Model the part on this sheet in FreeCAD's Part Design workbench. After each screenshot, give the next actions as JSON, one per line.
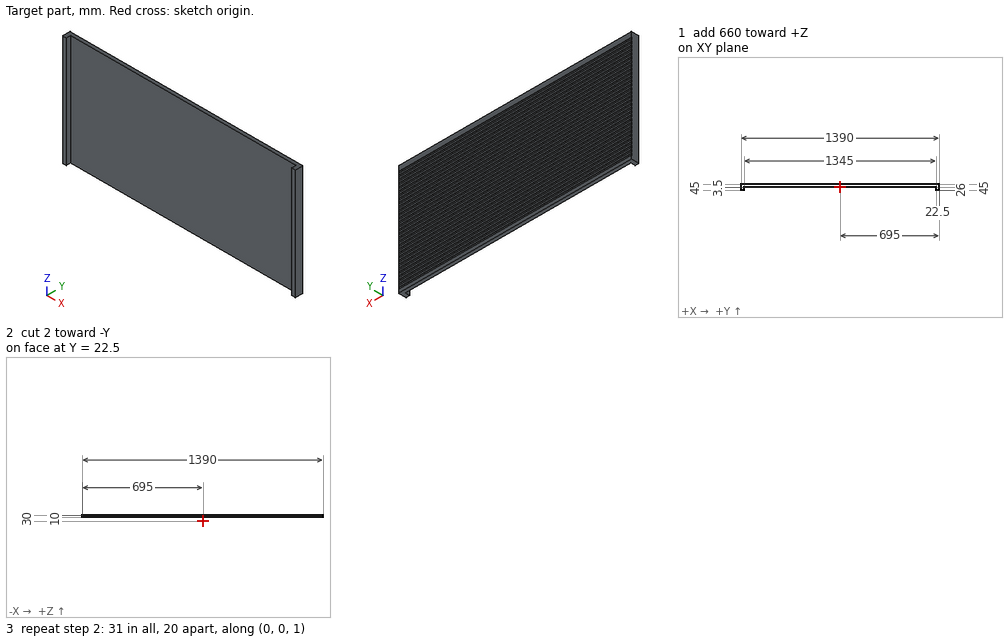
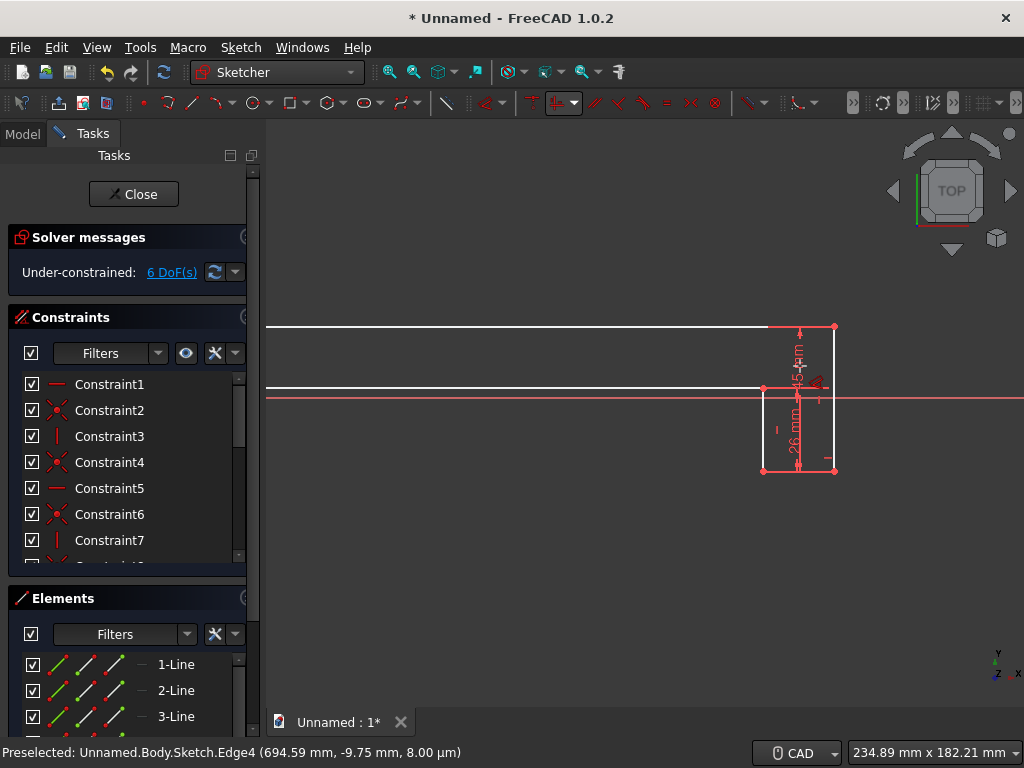
{"action": "scroll", "coordinate": [774, 415], "scroll_direction": "down", "scroll_amount": 12}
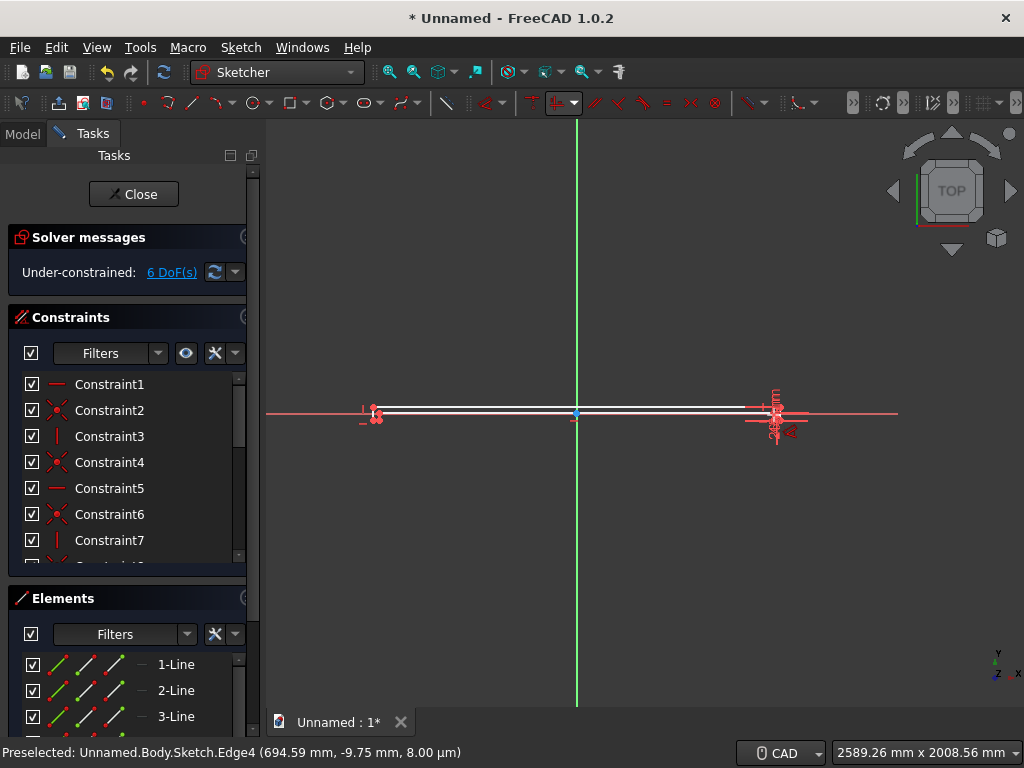
{"action": "scroll", "coordinate": [373, 411], "scroll_direction": "up", "scroll_amount": 9}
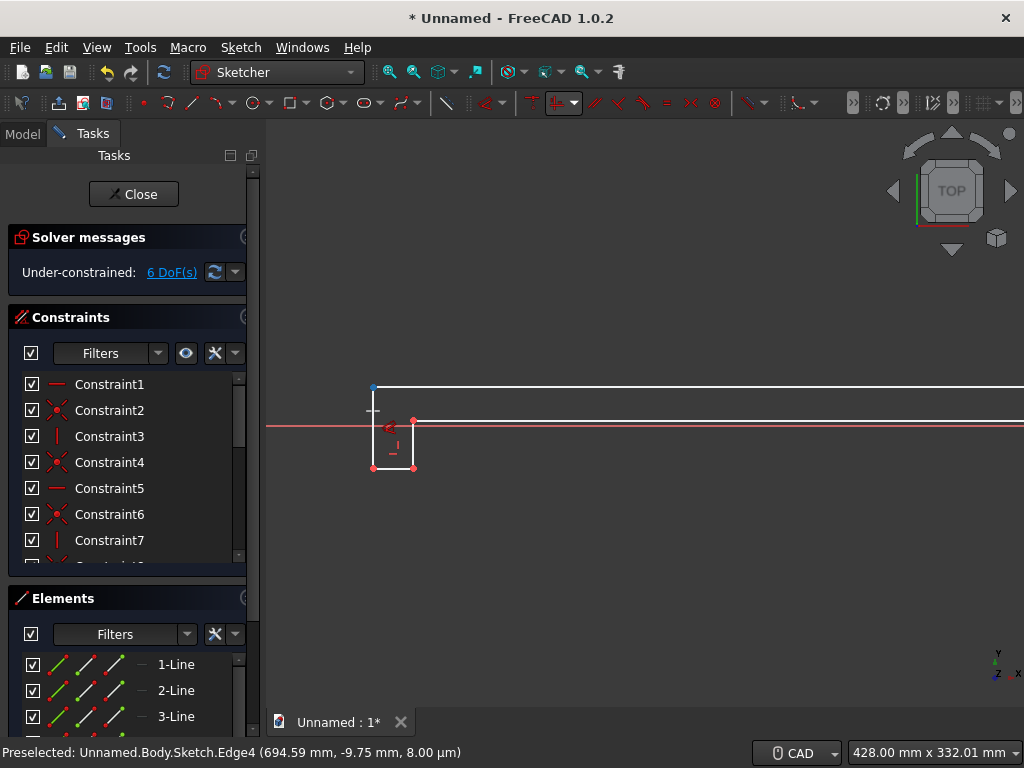
{"action": "left_click", "coordinate": [373, 412]}
{"action": "left_click", "coordinate": [339, 409]}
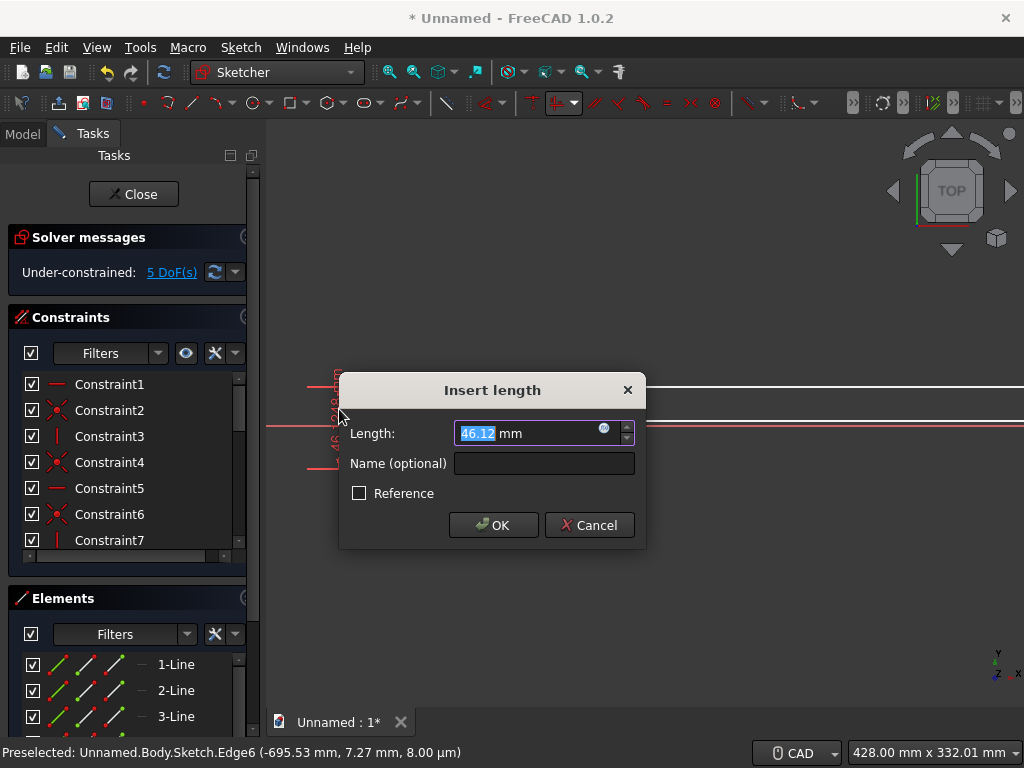
{"action": "type", "text": "45"}
{"action": "key", "text": "Return"}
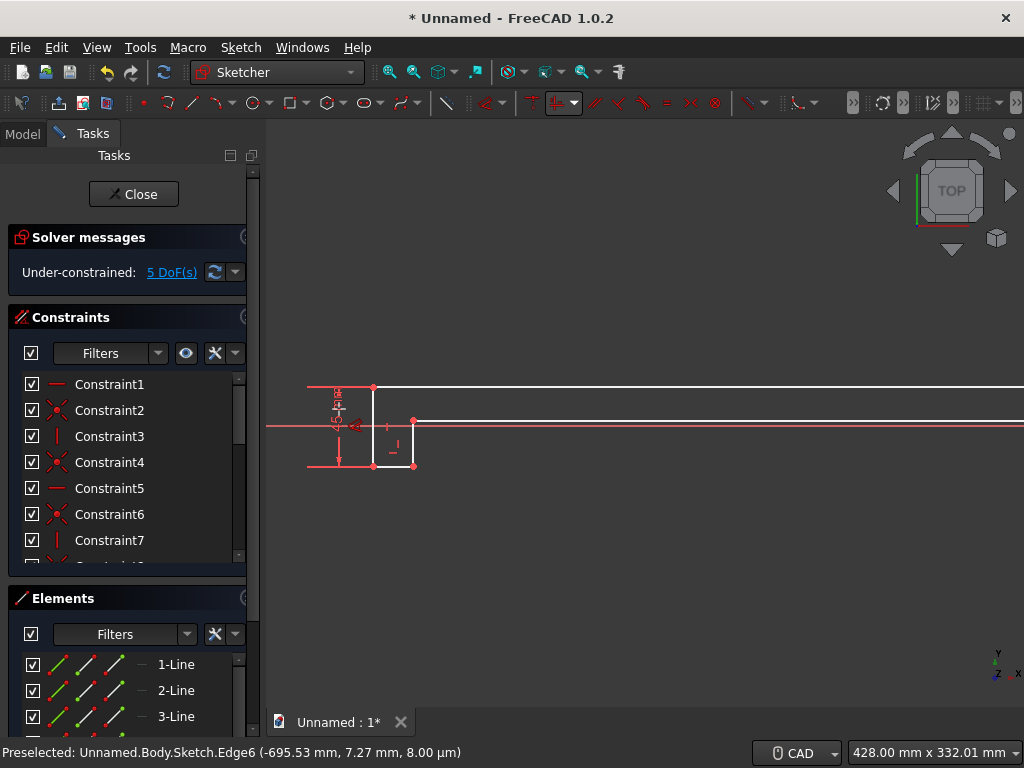
{"action": "scroll", "coordinate": [373, 410], "scroll_direction": "down", "scroll_amount": 9}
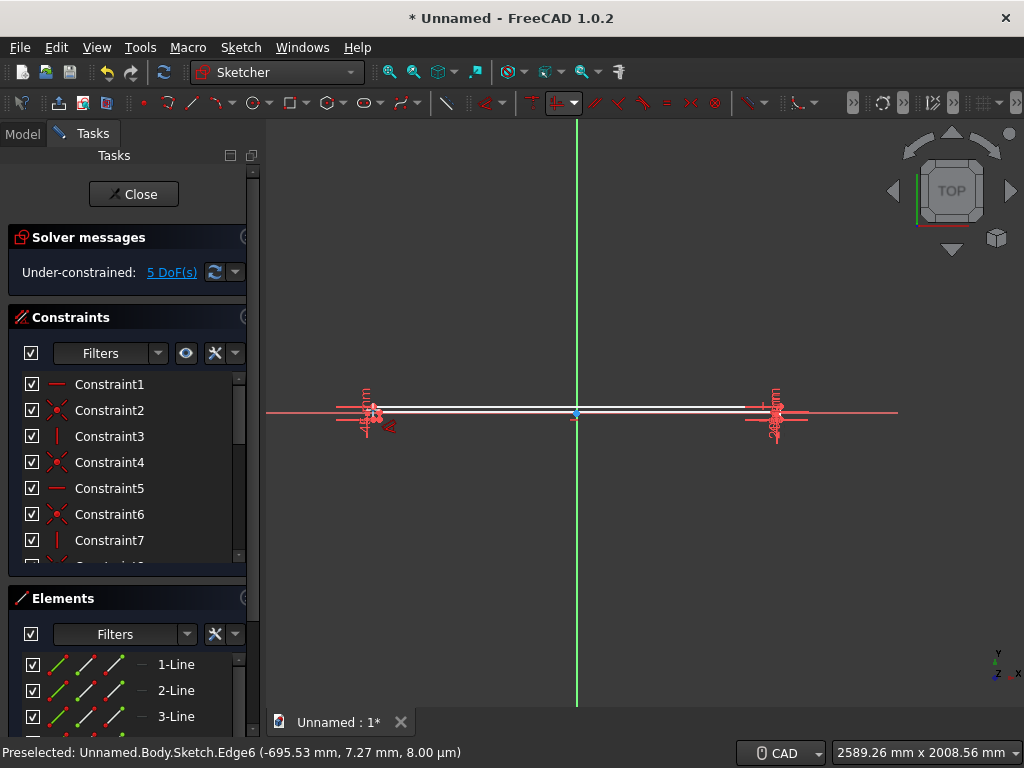
{"action": "scroll", "coordinate": [498, 412], "scroll_direction": "up", "scroll_amount": 14}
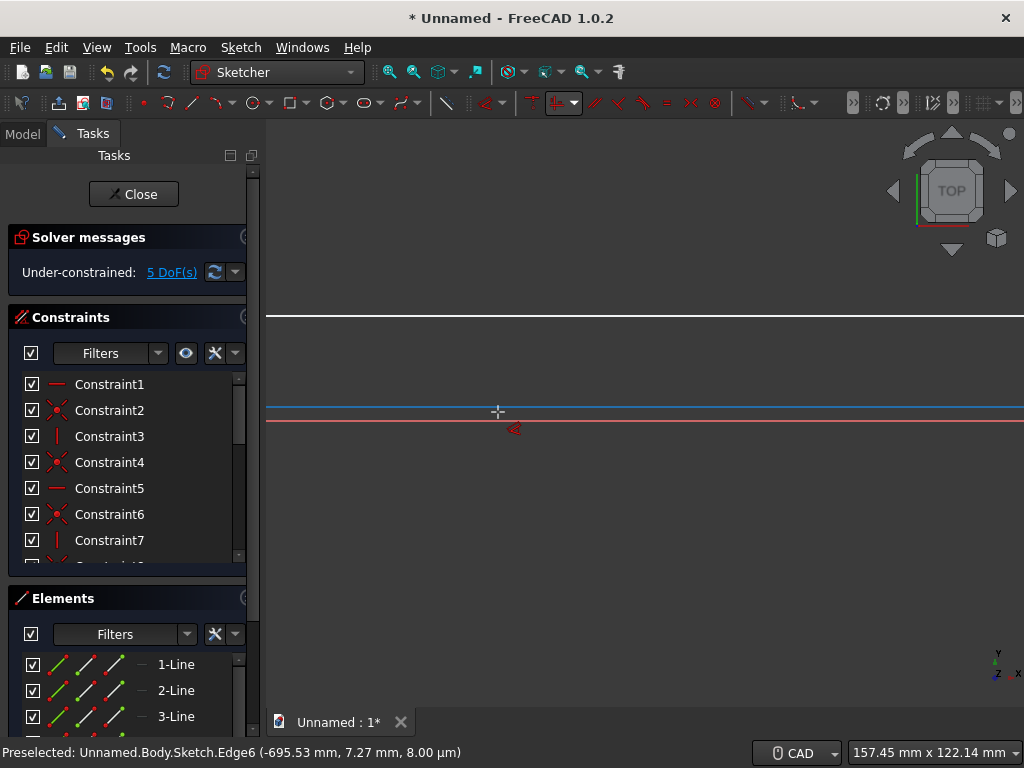
{"action": "left_click", "coordinate": [492, 407]}
{"action": "left_click", "coordinate": [576, 373]}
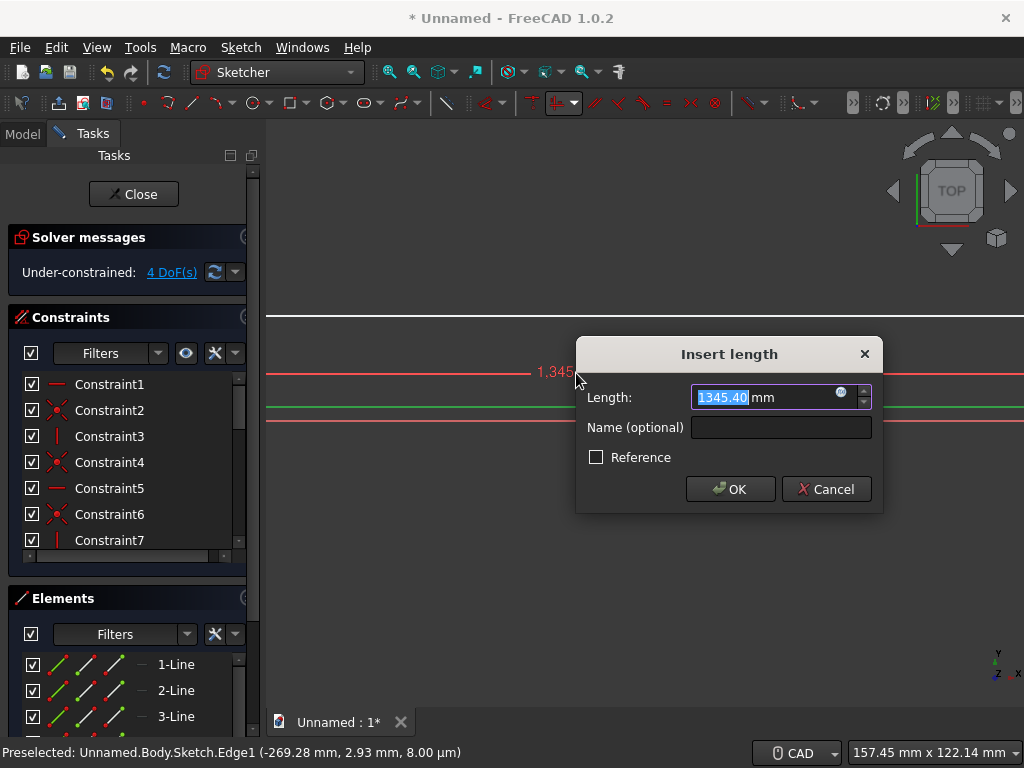
{"action": "type", "text": "1345"}
{"action": "key", "text": "Return"}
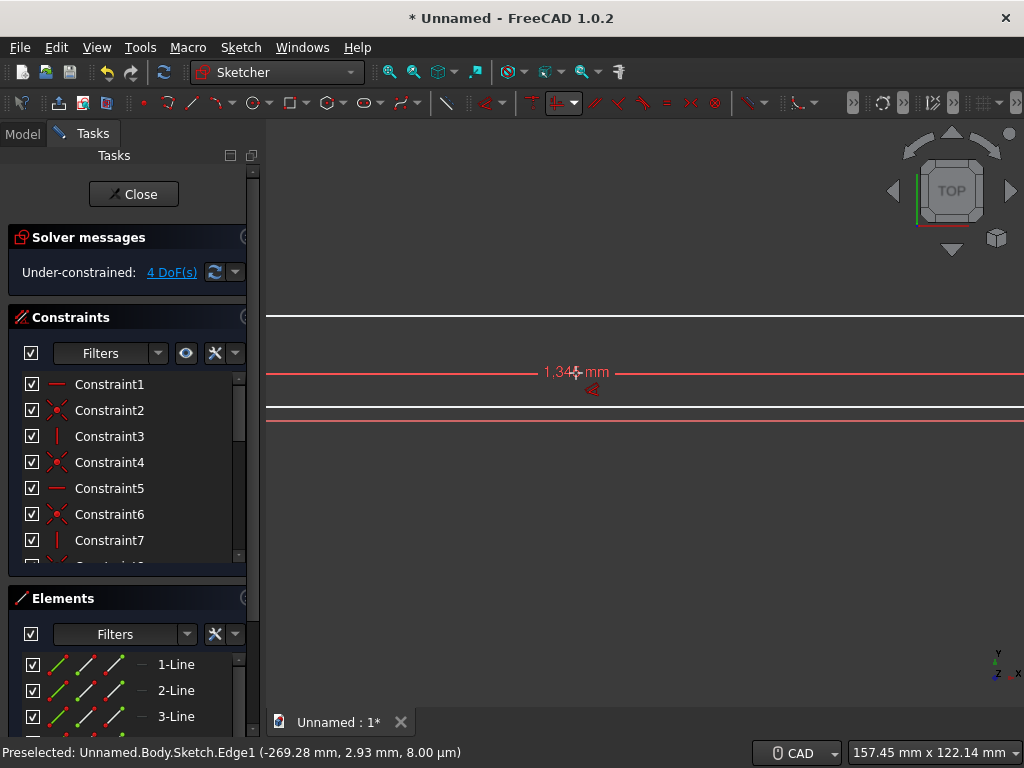
{"action": "scroll", "coordinate": [498, 412], "scroll_direction": "down", "scroll_amount": 14}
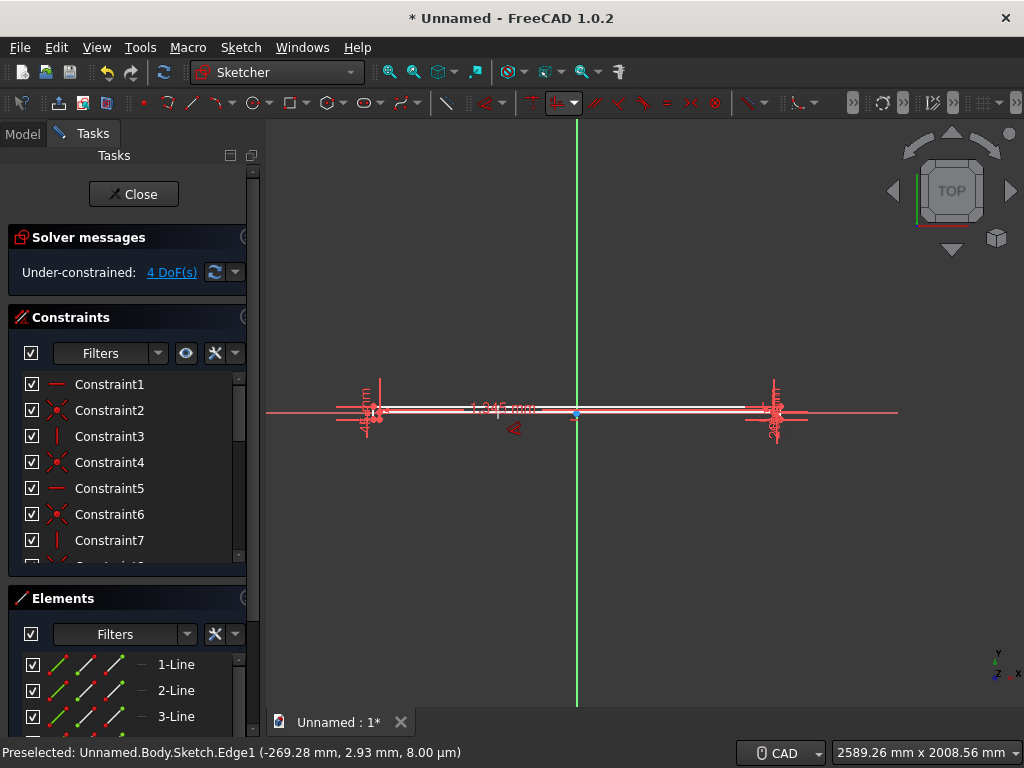
{"action": "scroll", "coordinate": [776, 420], "scroll_direction": "up", "scroll_amount": 10}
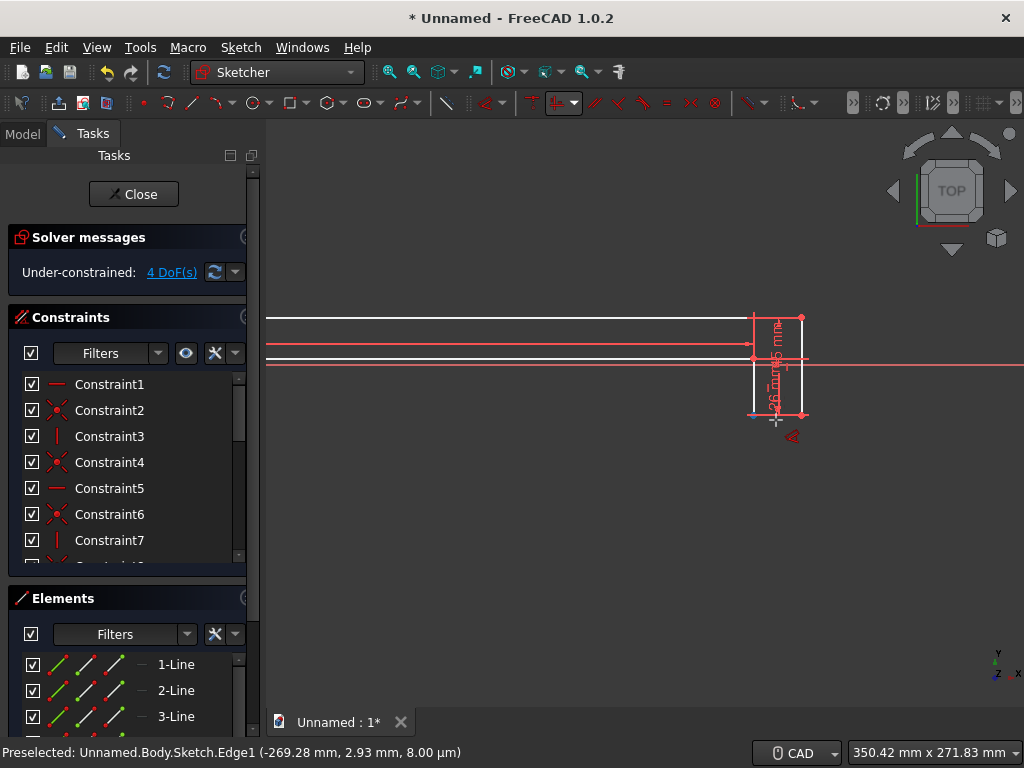
{"action": "left_click", "coordinate": [768, 415]}
{"action": "left_click", "coordinate": [778, 449]}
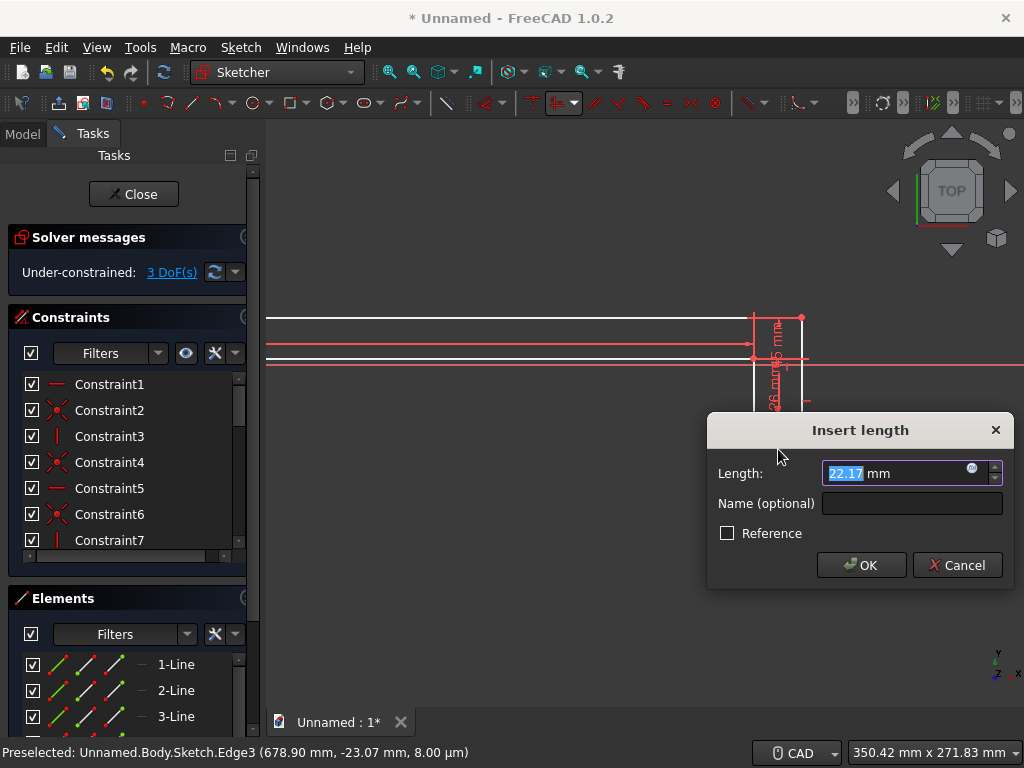
{"action": "type", "text": "22.5"}
{"action": "key", "text": "Return"}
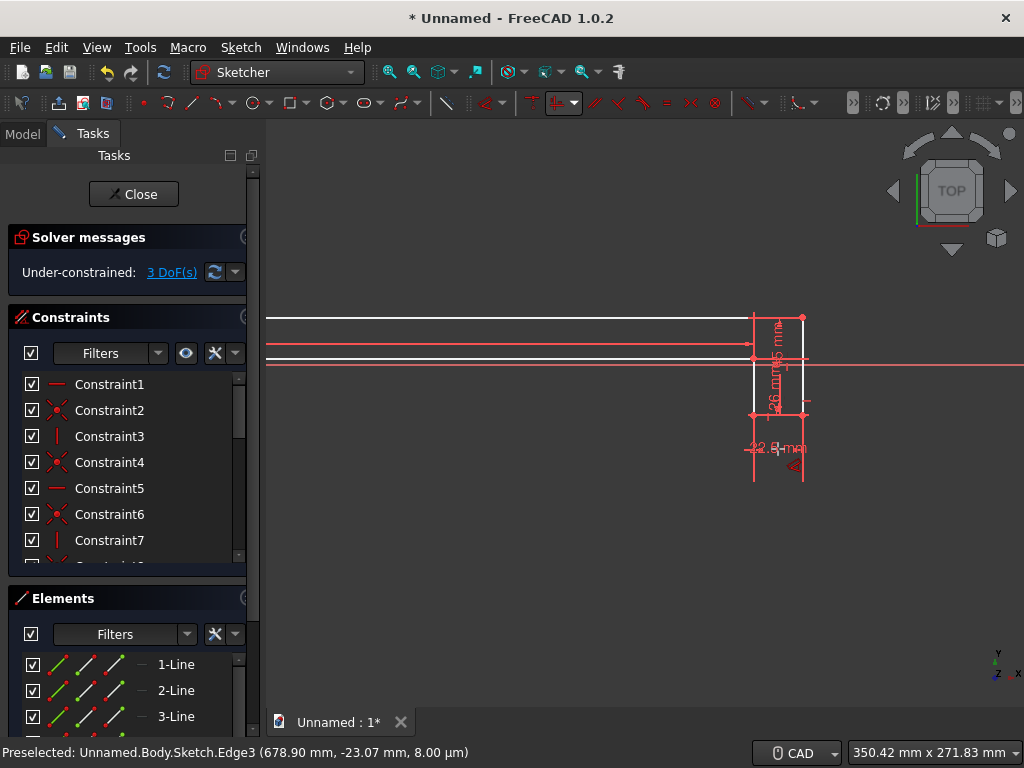
{"action": "scroll", "coordinate": [776, 420], "scroll_direction": "down", "scroll_amount": 10}